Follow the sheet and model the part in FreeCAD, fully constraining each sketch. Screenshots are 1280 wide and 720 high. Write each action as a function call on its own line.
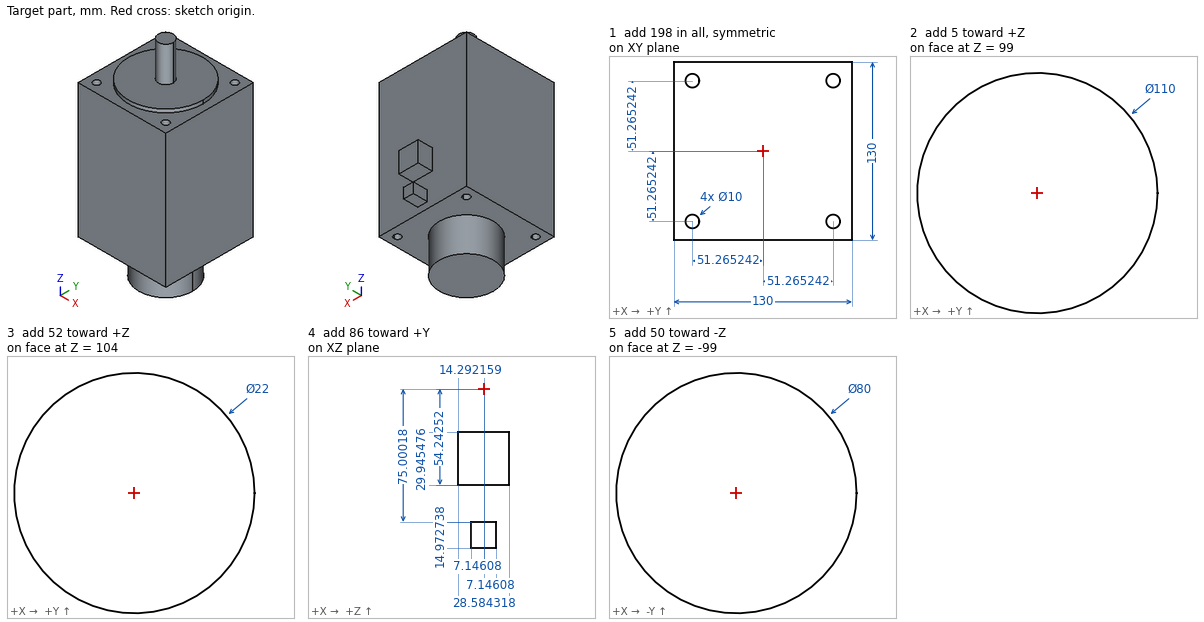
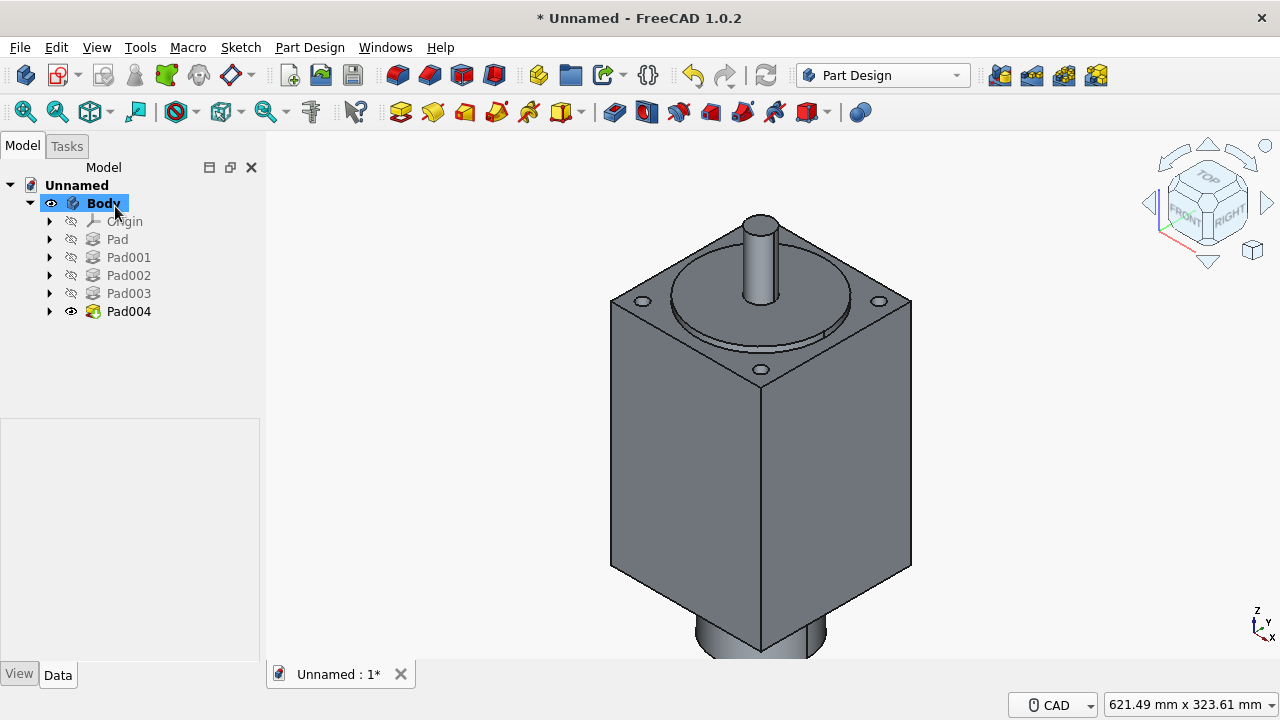
key(v)
key(f)